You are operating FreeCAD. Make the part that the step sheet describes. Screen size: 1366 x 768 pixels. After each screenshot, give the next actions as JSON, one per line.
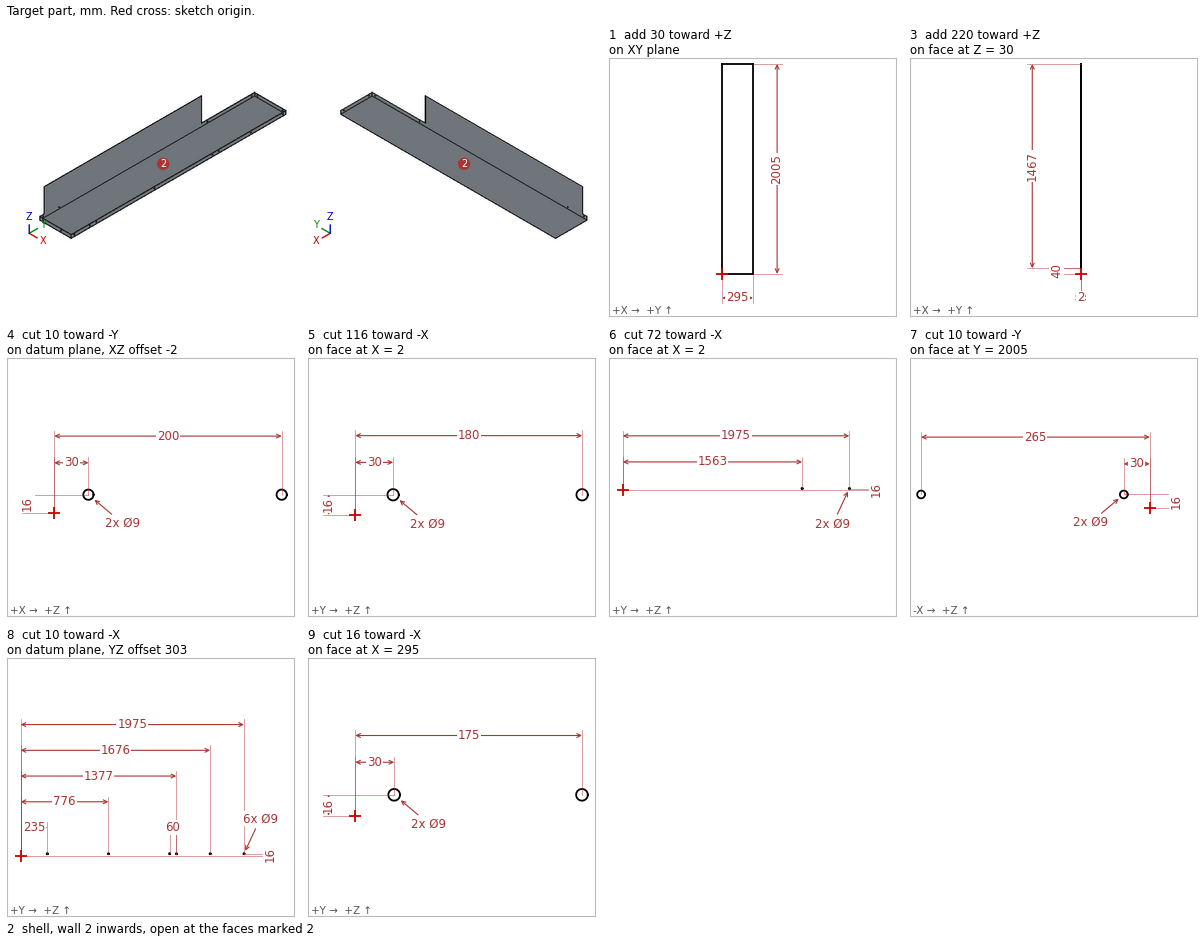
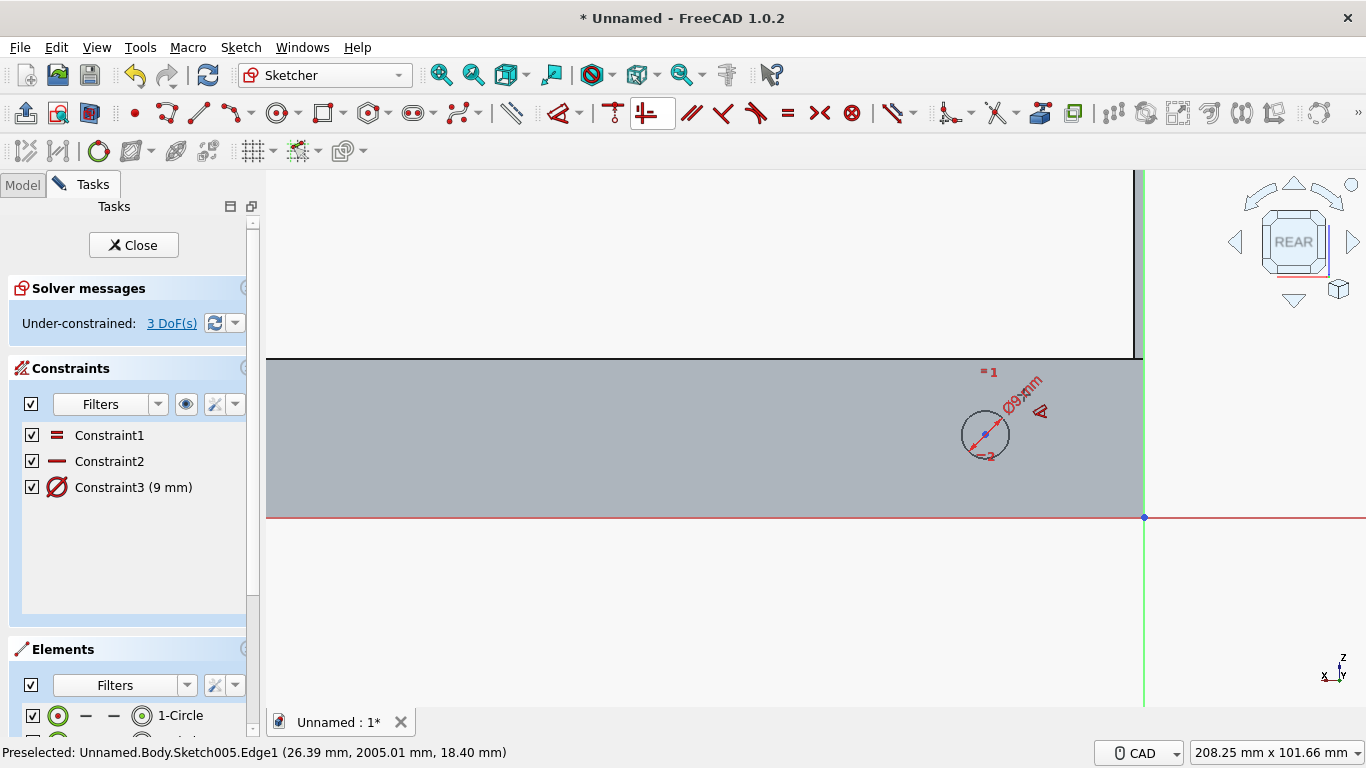
{"action": "left_click", "coordinate": [985, 435]}
{"action": "left_click", "coordinate": [1065, 552]}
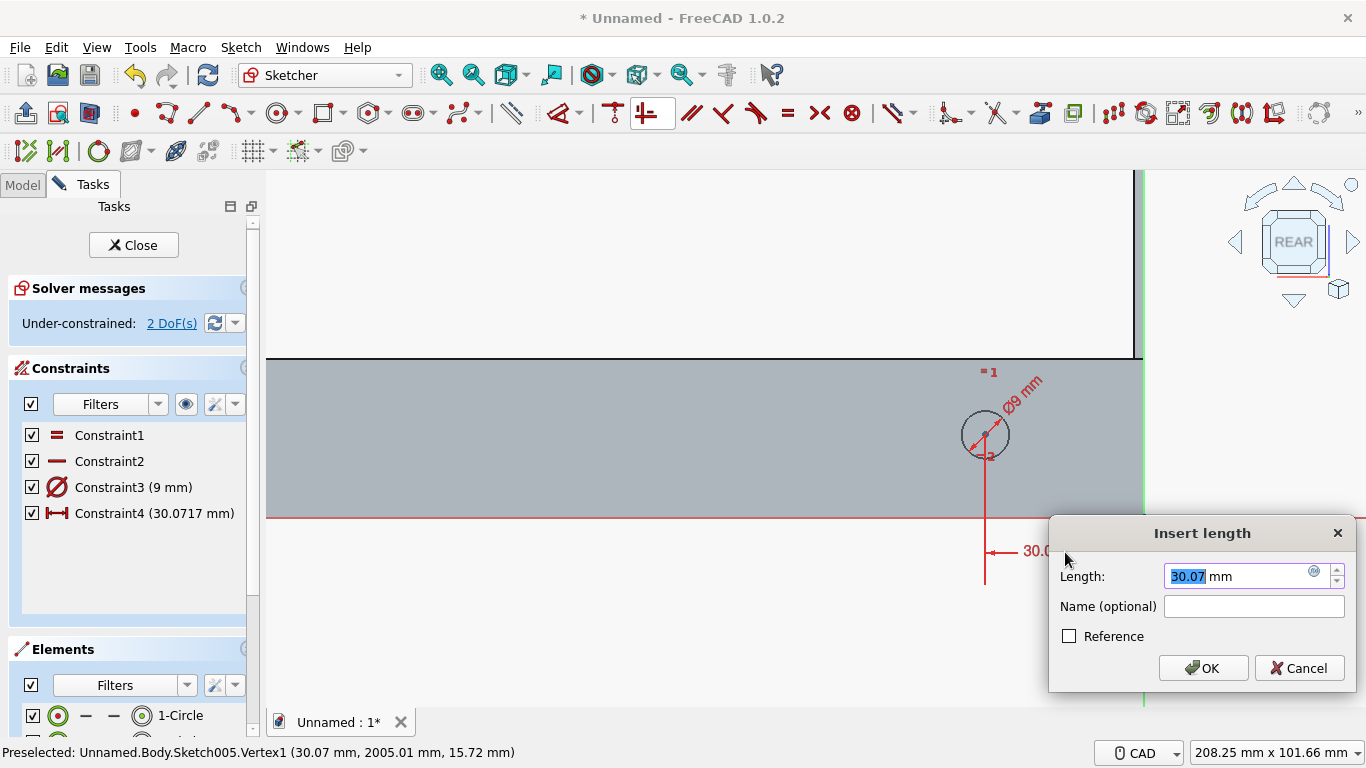
{"action": "type", "text": "30"}
{"action": "key", "text": "Return"}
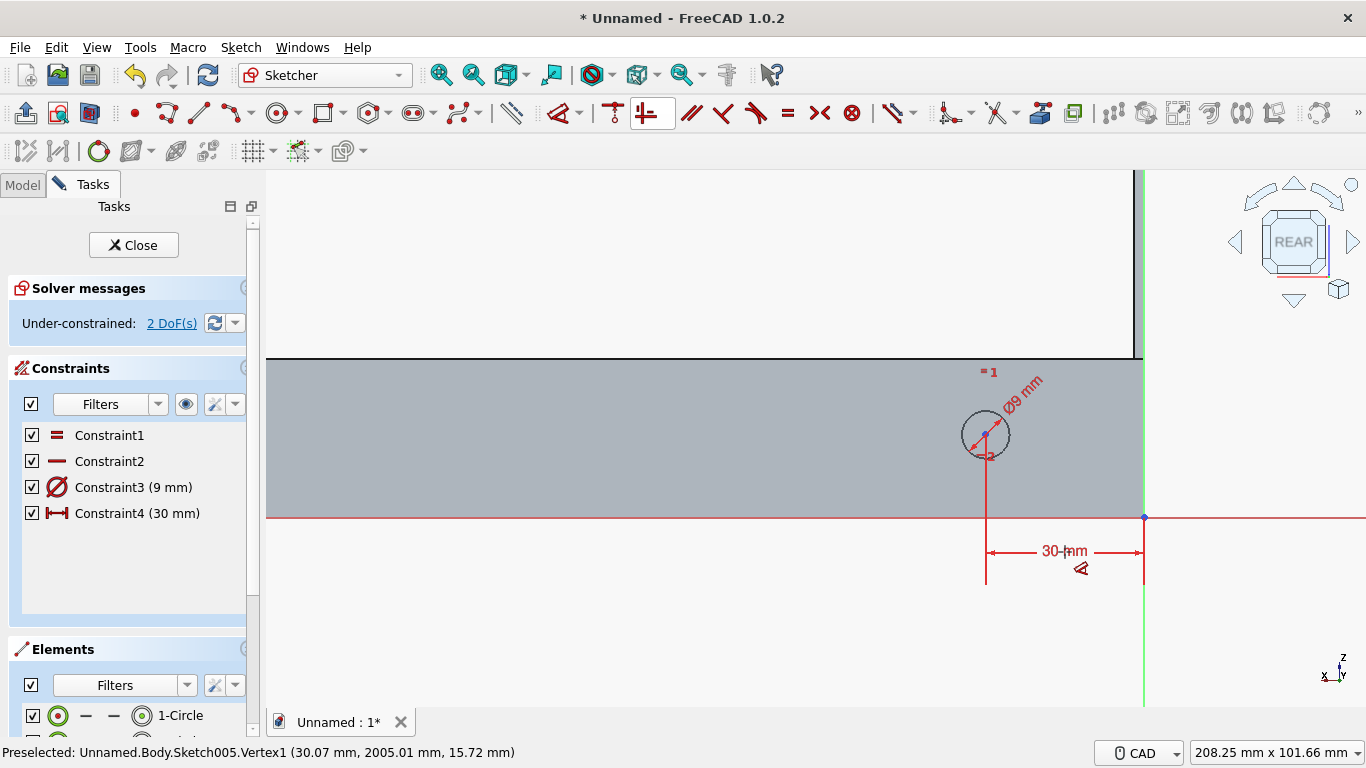
{"action": "left_click", "coordinate": [986, 435]}
{"action": "left_click", "coordinate": [1178, 476]}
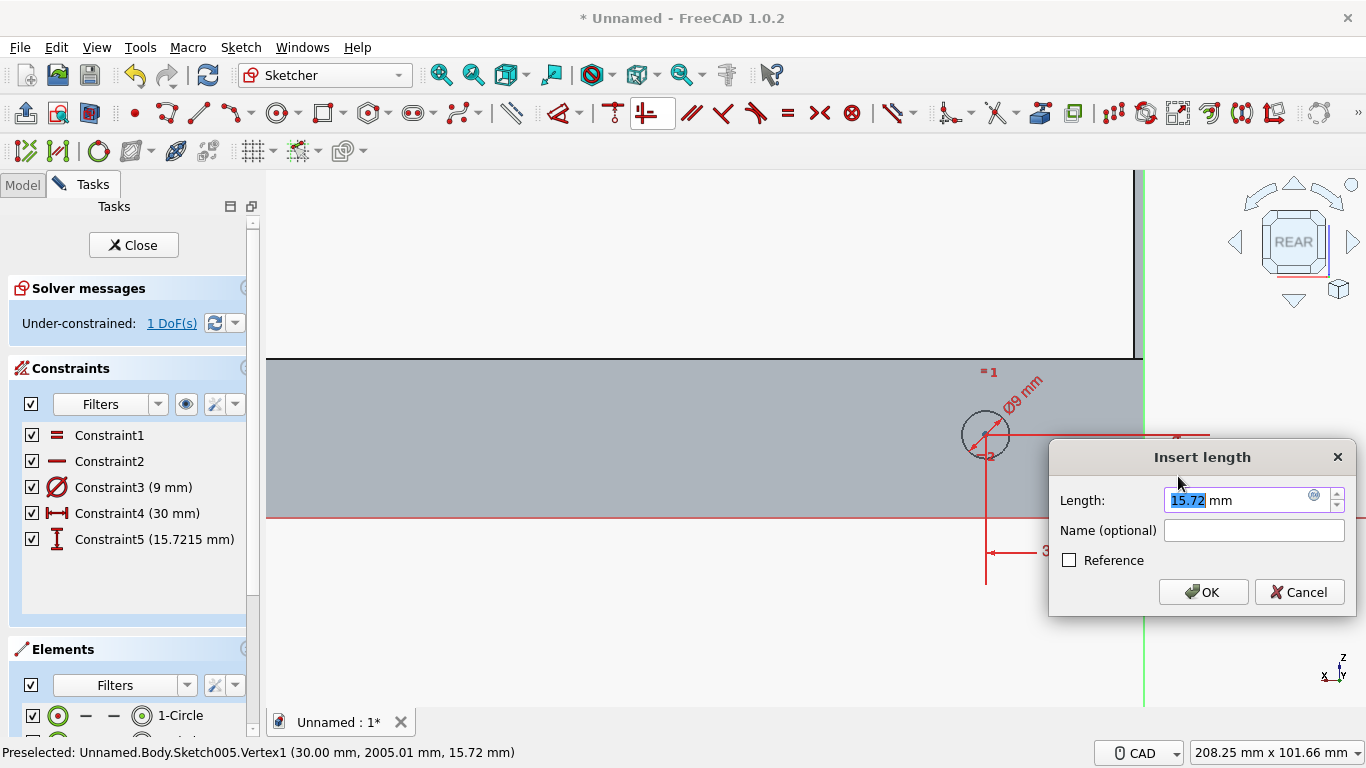
{"action": "type", "text": "16"}
{"action": "key", "text": "Return"}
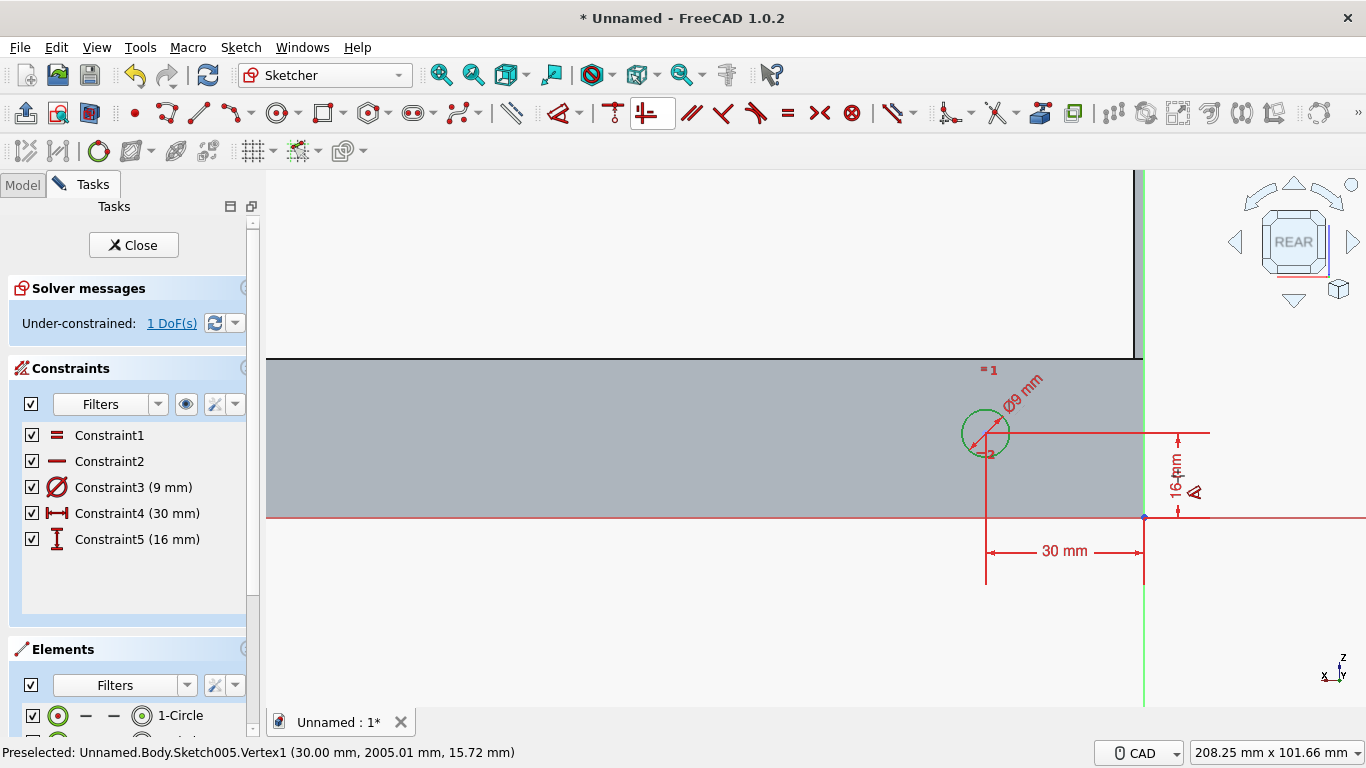
{"action": "scroll", "coordinate": [1005, 418], "scroll_direction": "down", "scroll_amount": 4}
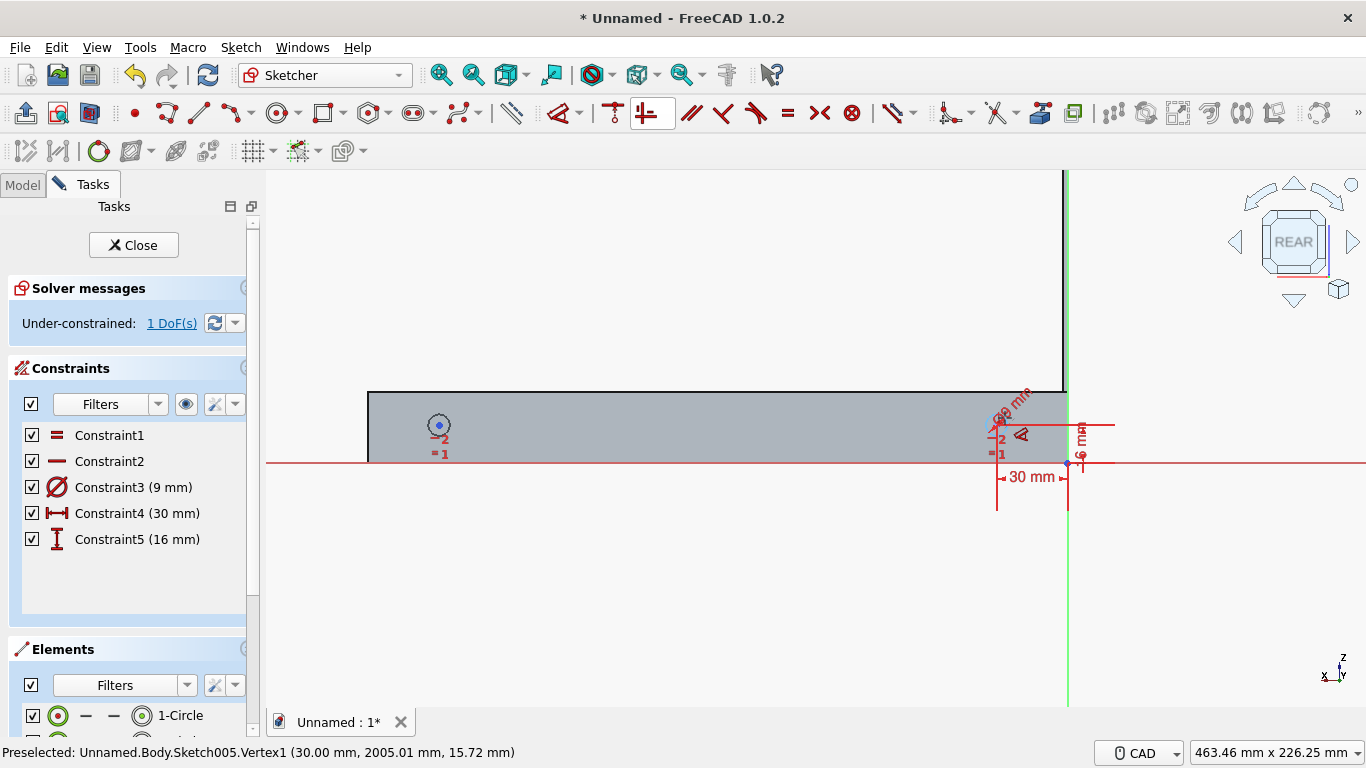
{"action": "left_click", "coordinate": [439, 425]}
{"action": "left_click", "coordinate": [754, 497]}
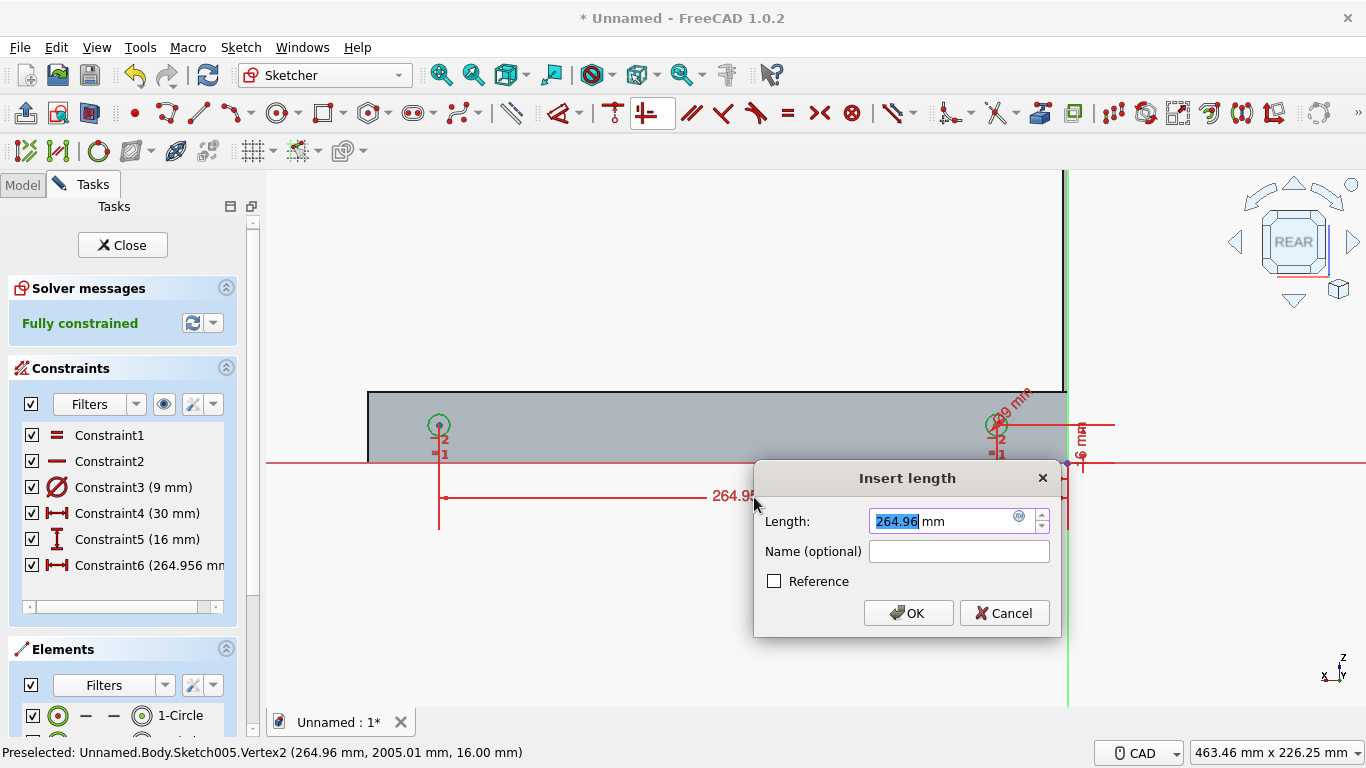
{"action": "type", "text": "265"}
{"action": "key", "text": "Return"}
{"action": "key", "text": "Escape"}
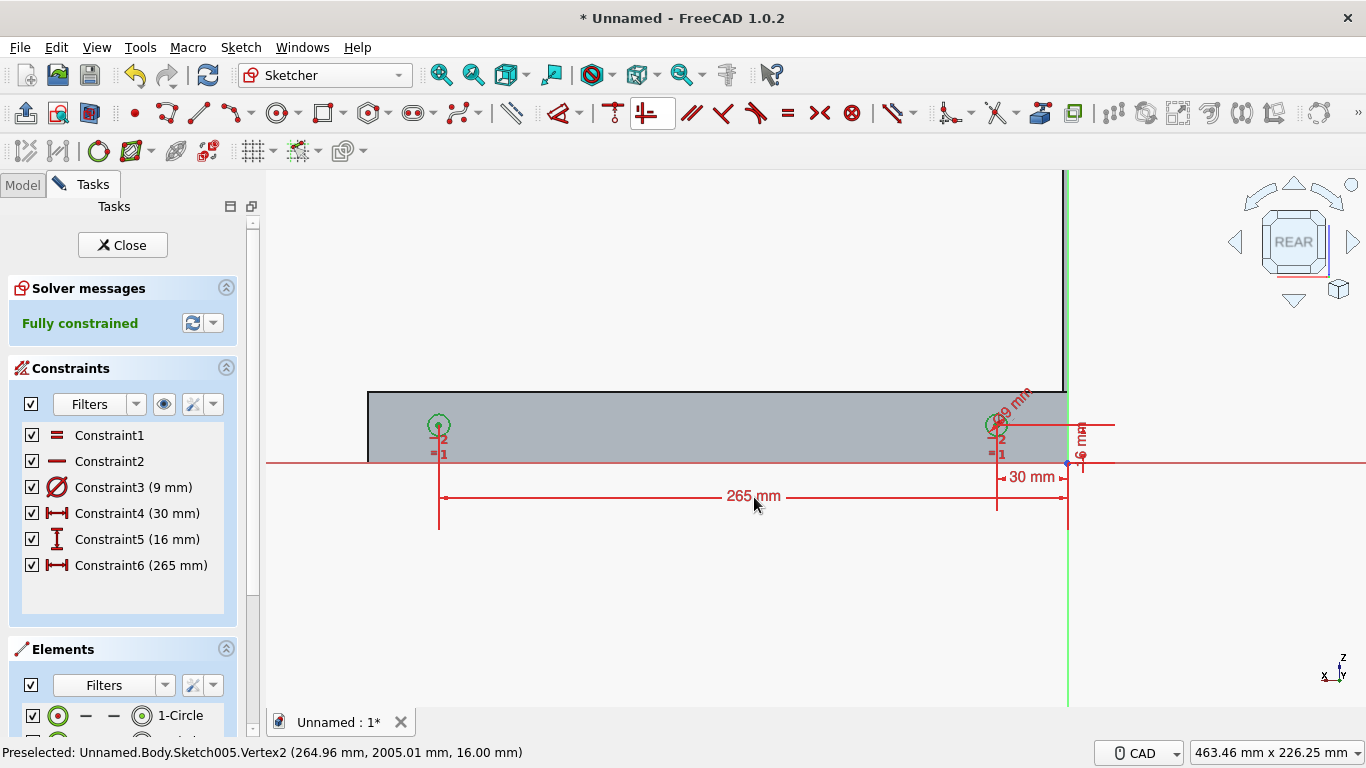
{"action": "left_click", "coordinate": [123, 245]}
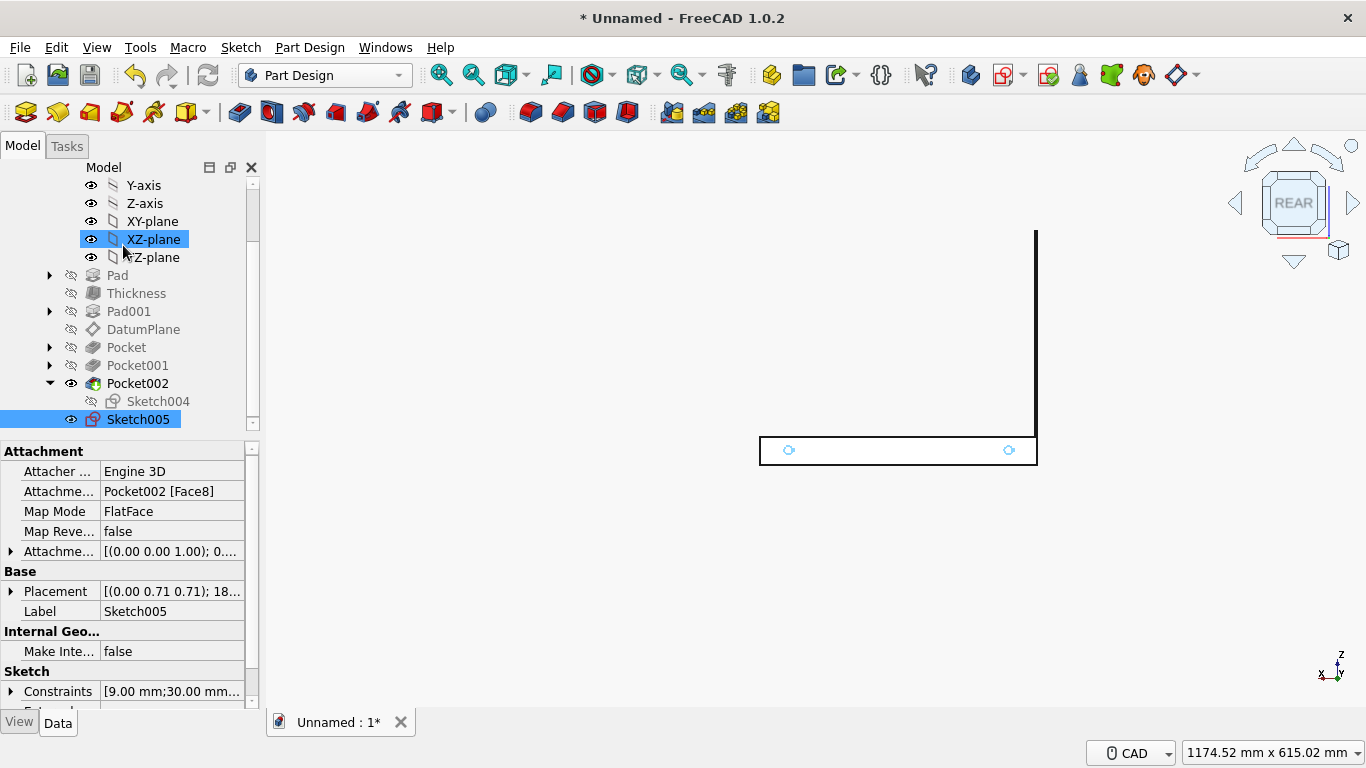
{"action": "left_click", "coordinate": [240, 112]}